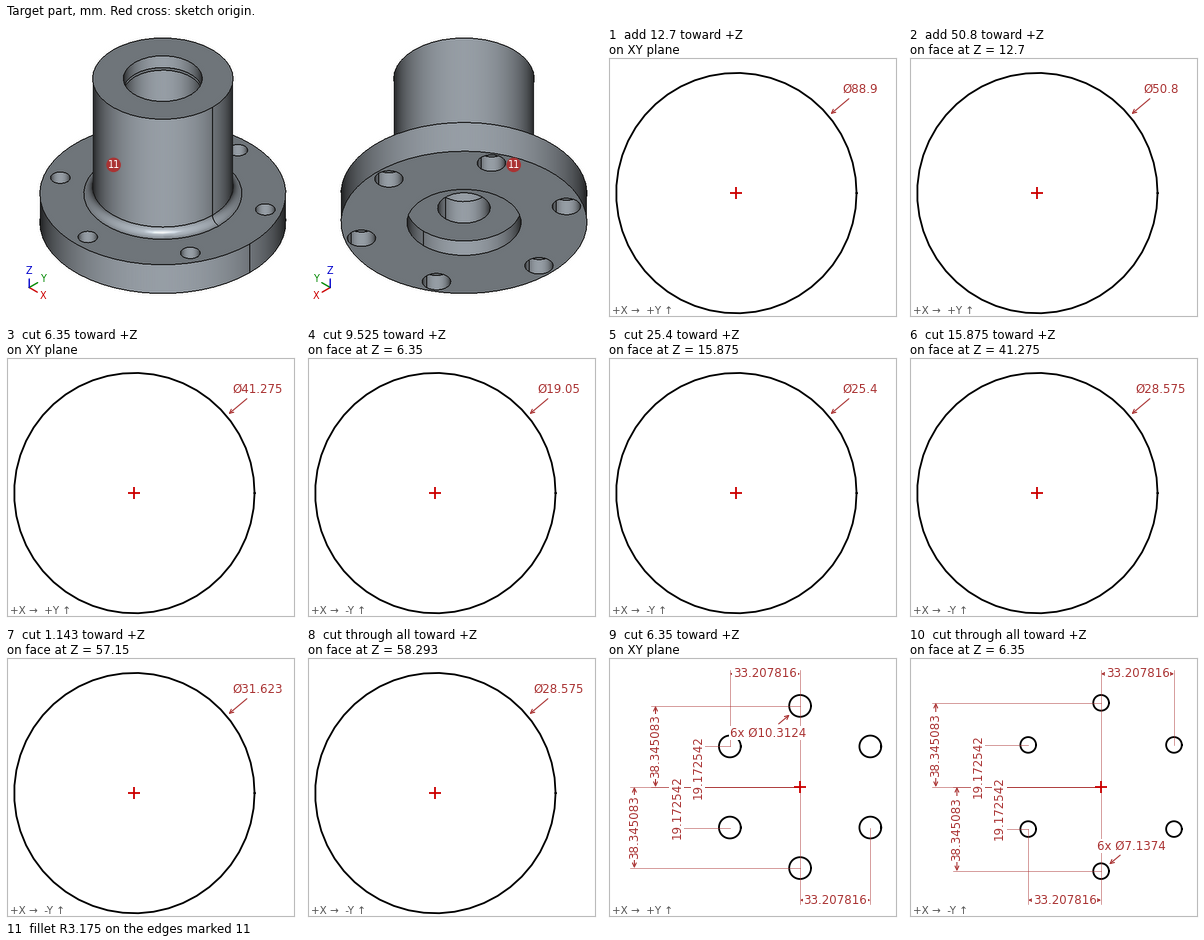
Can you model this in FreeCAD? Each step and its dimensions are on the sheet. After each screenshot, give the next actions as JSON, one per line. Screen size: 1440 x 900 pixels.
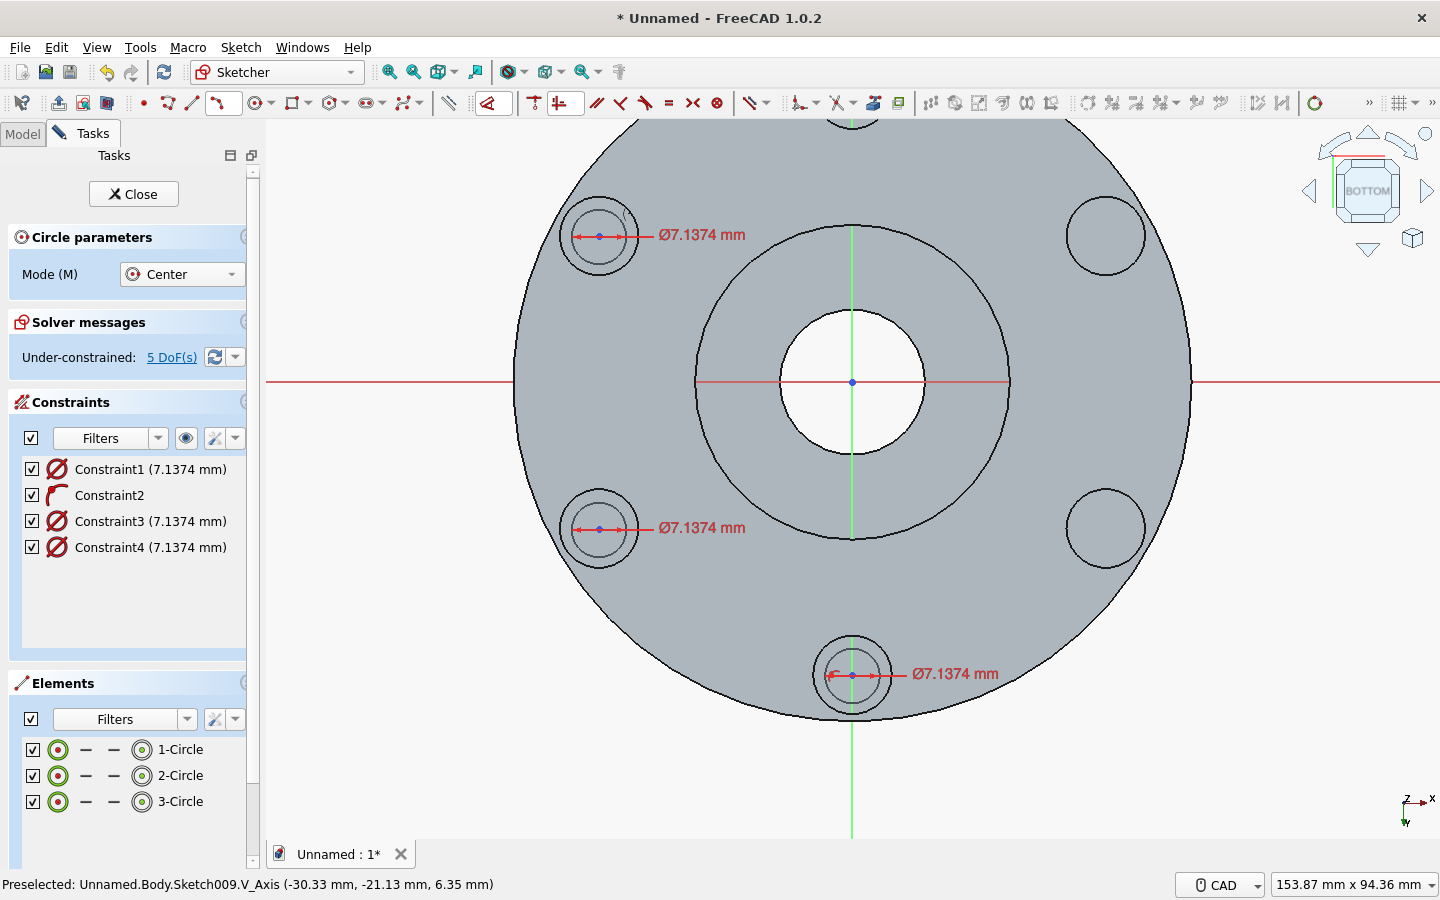
{"action": "scroll", "coordinate": [646, 676], "scroll_direction": "down", "scroll_amount": 2}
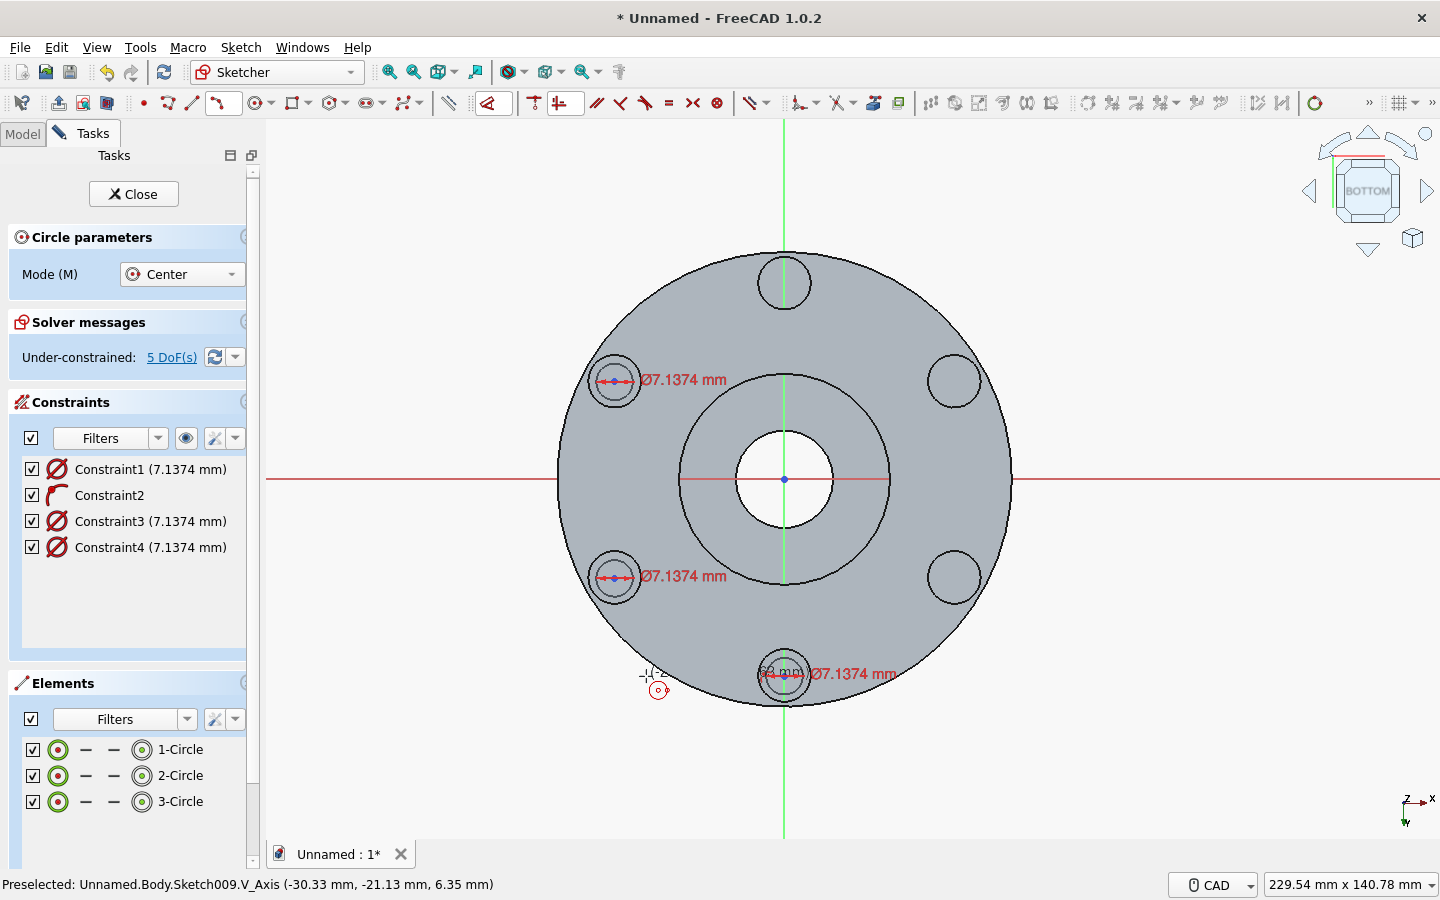
{"action": "scroll", "coordinate": [784, 283], "scroll_direction": "up", "scroll_amount": 2}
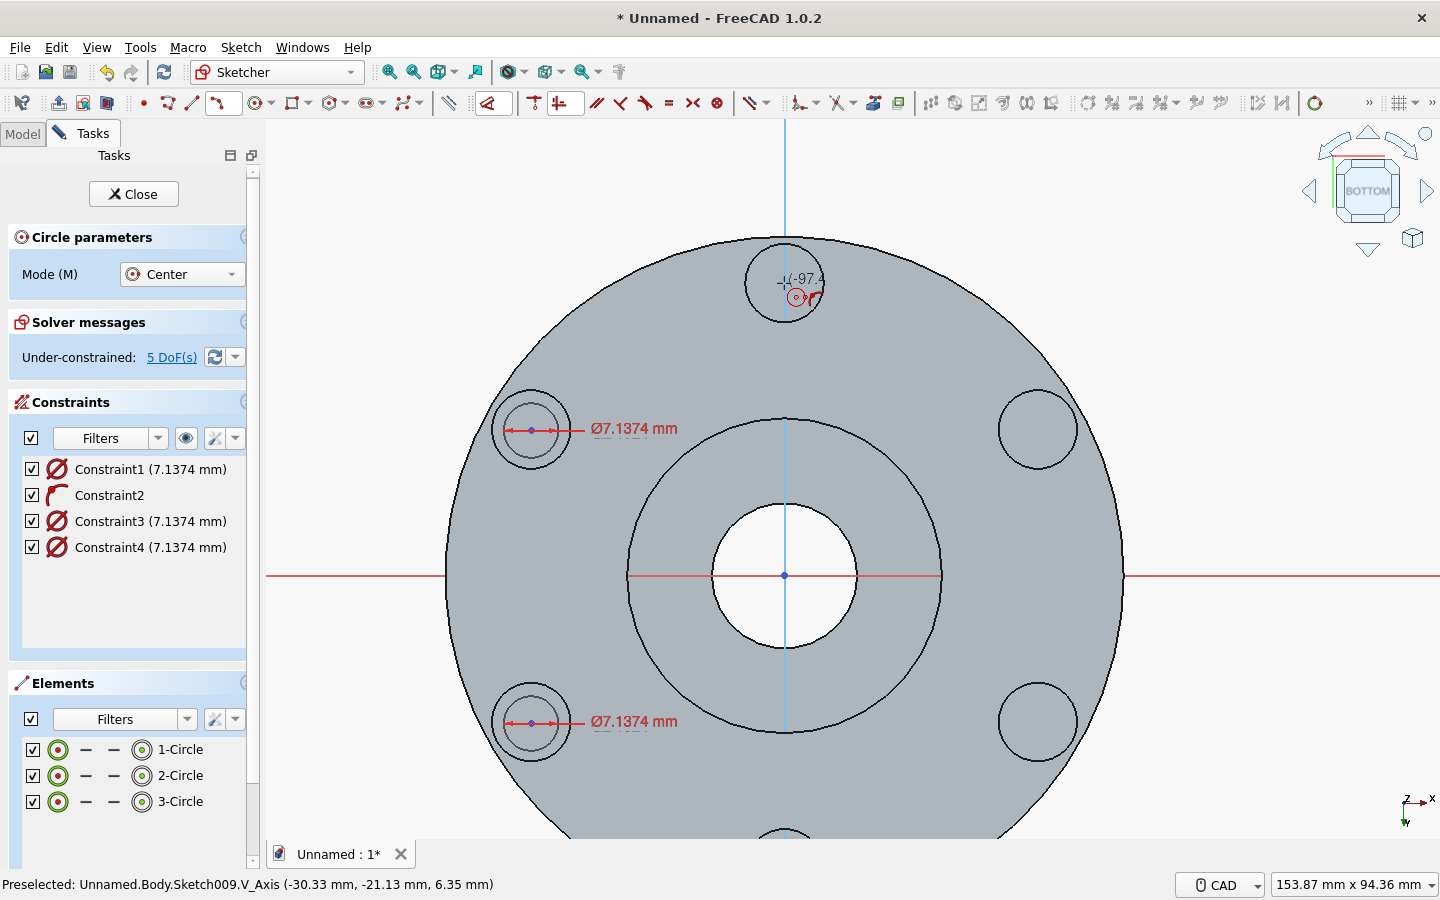
{"action": "left_click", "coordinate": [785, 283]}
{"action": "mouse_move", "coordinate": [804, 264]}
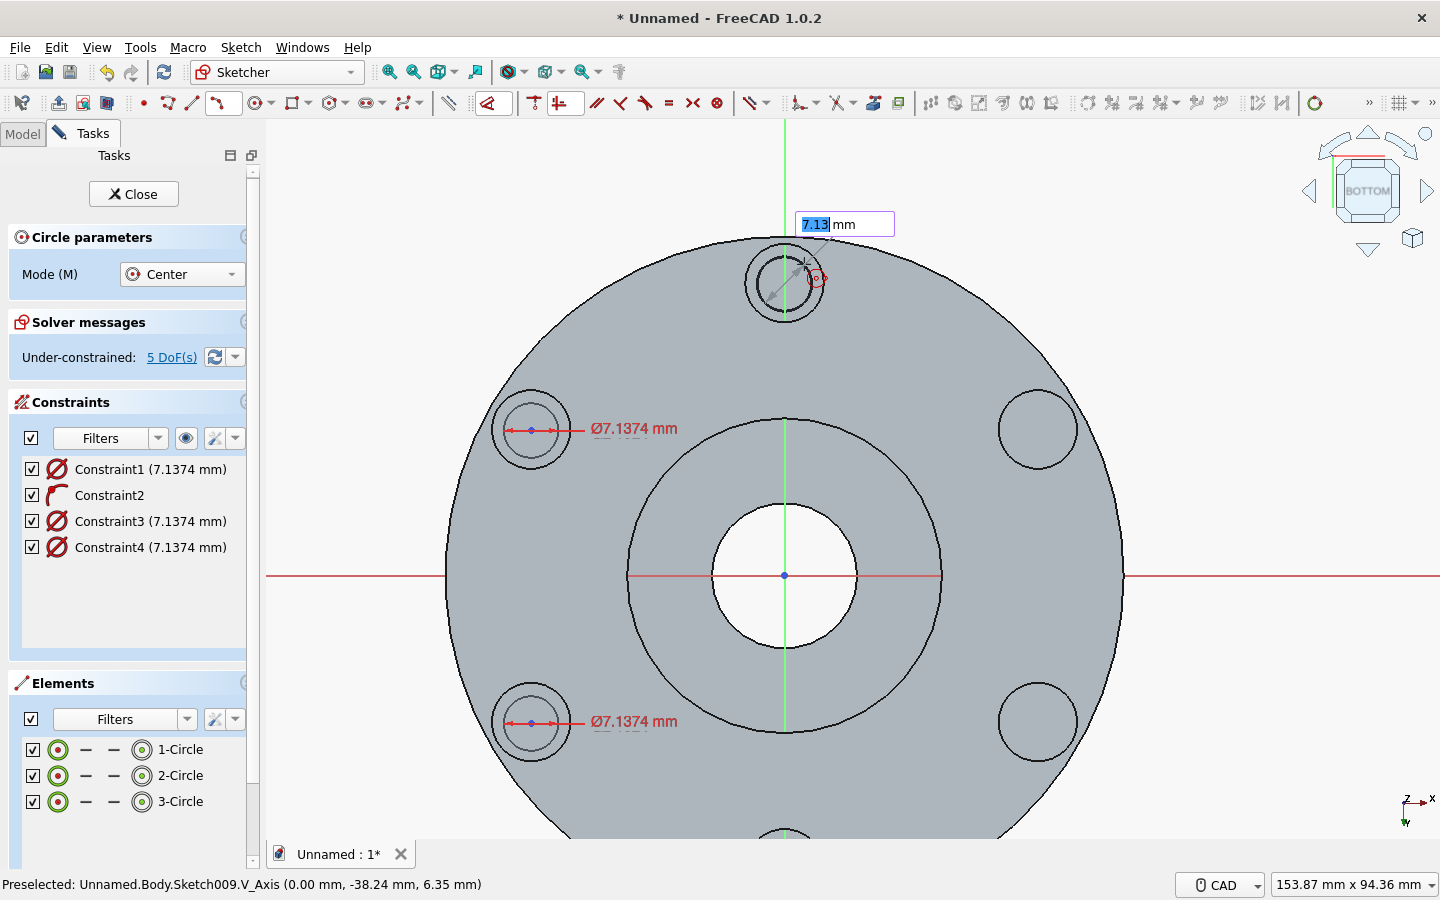
{"action": "type", "text": "7.1374"}
{"action": "key", "text": "Return"}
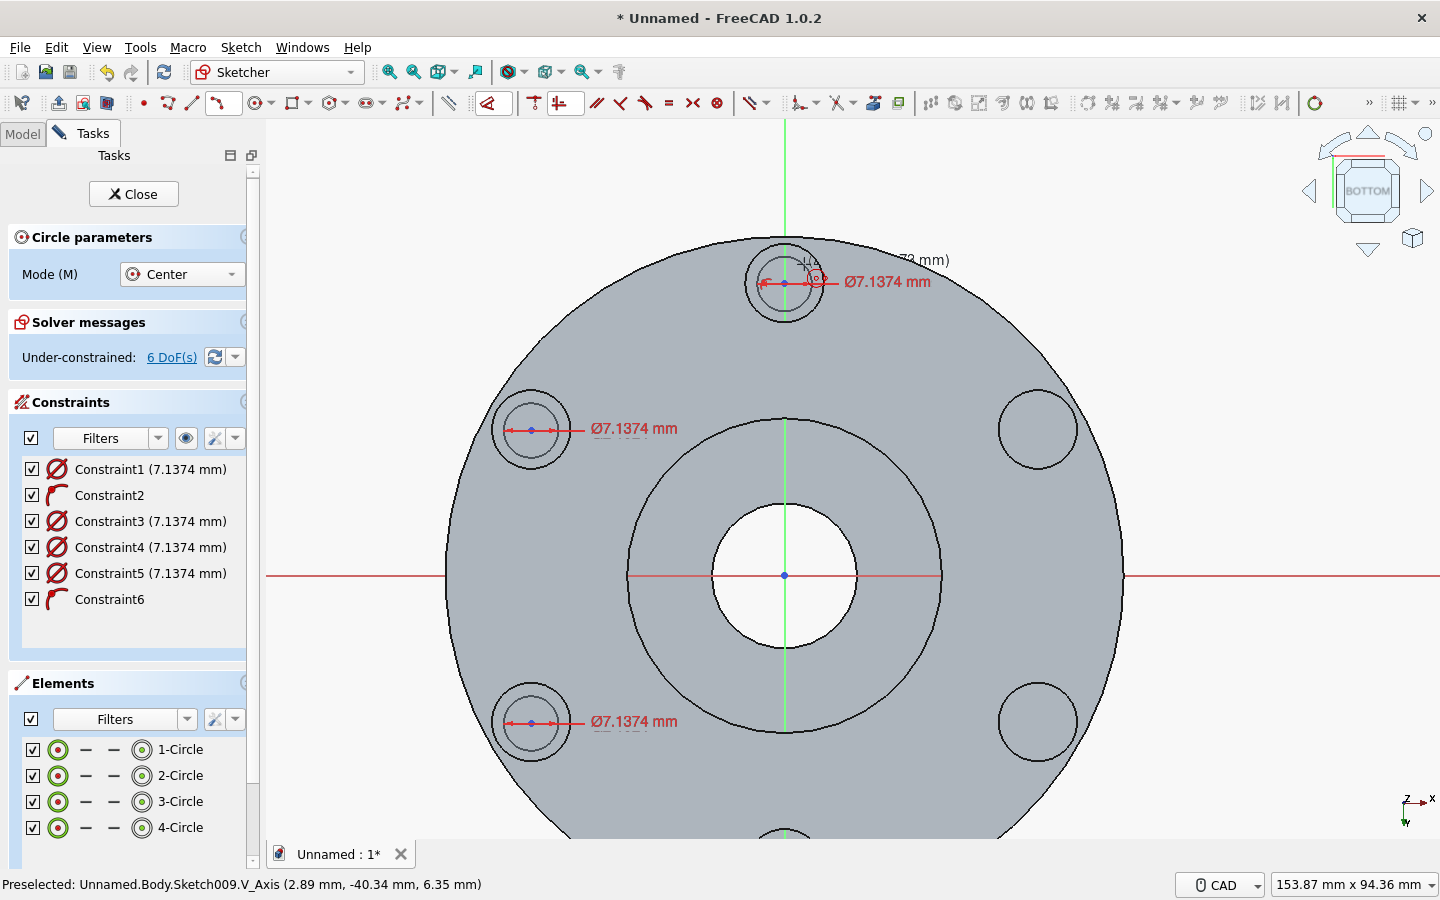
{"action": "left_click", "coordinate": [1038, 429]}
{"action": "mouse_move", "coordinate": [1057, 410]}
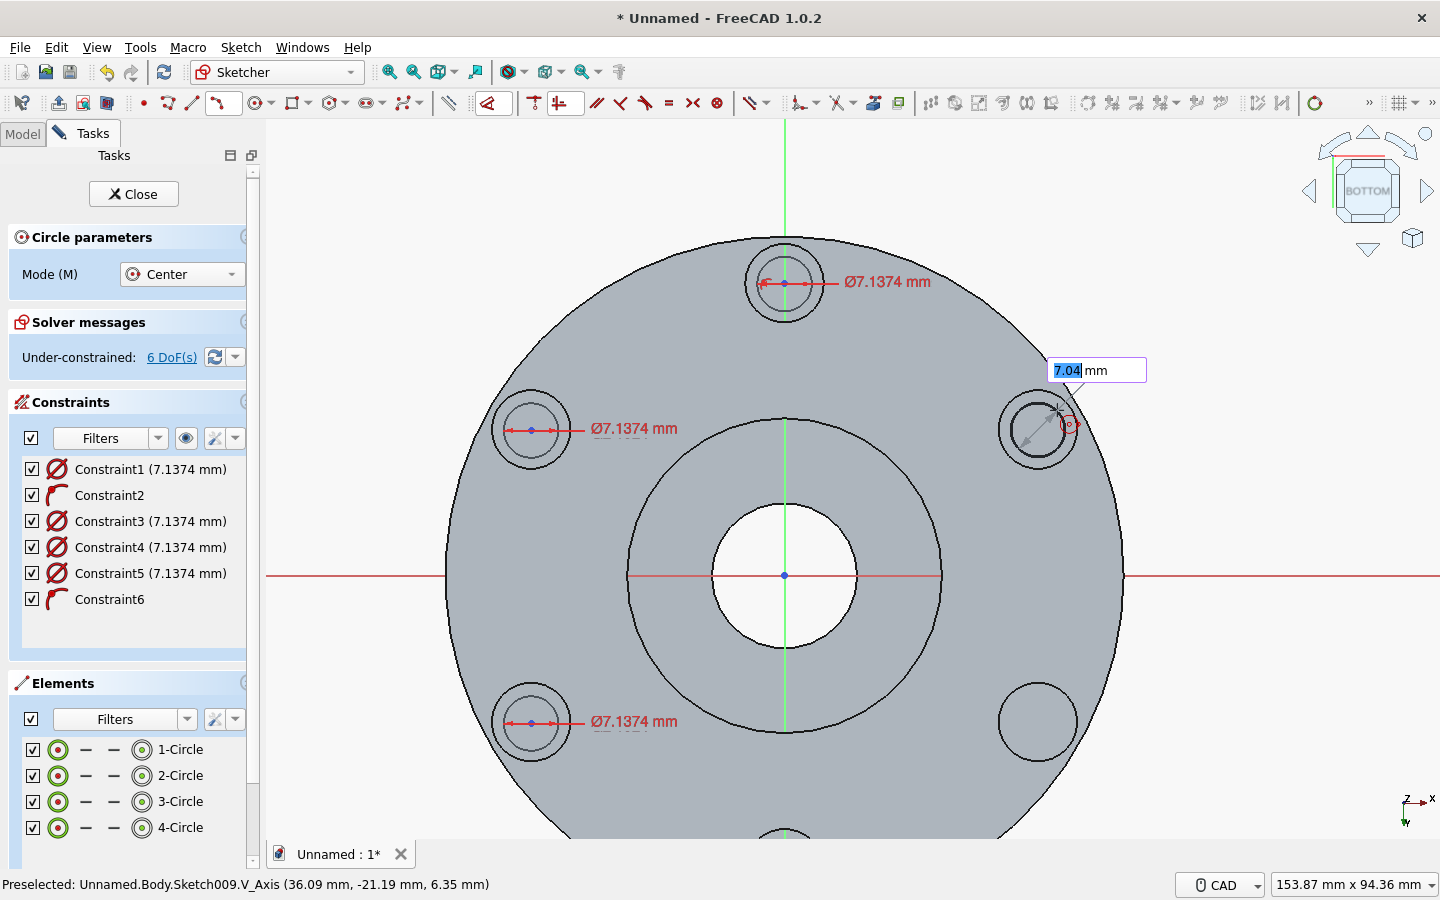
{"action": "type", "text": "7.1374"}
{"action": "key", "text": "Return"}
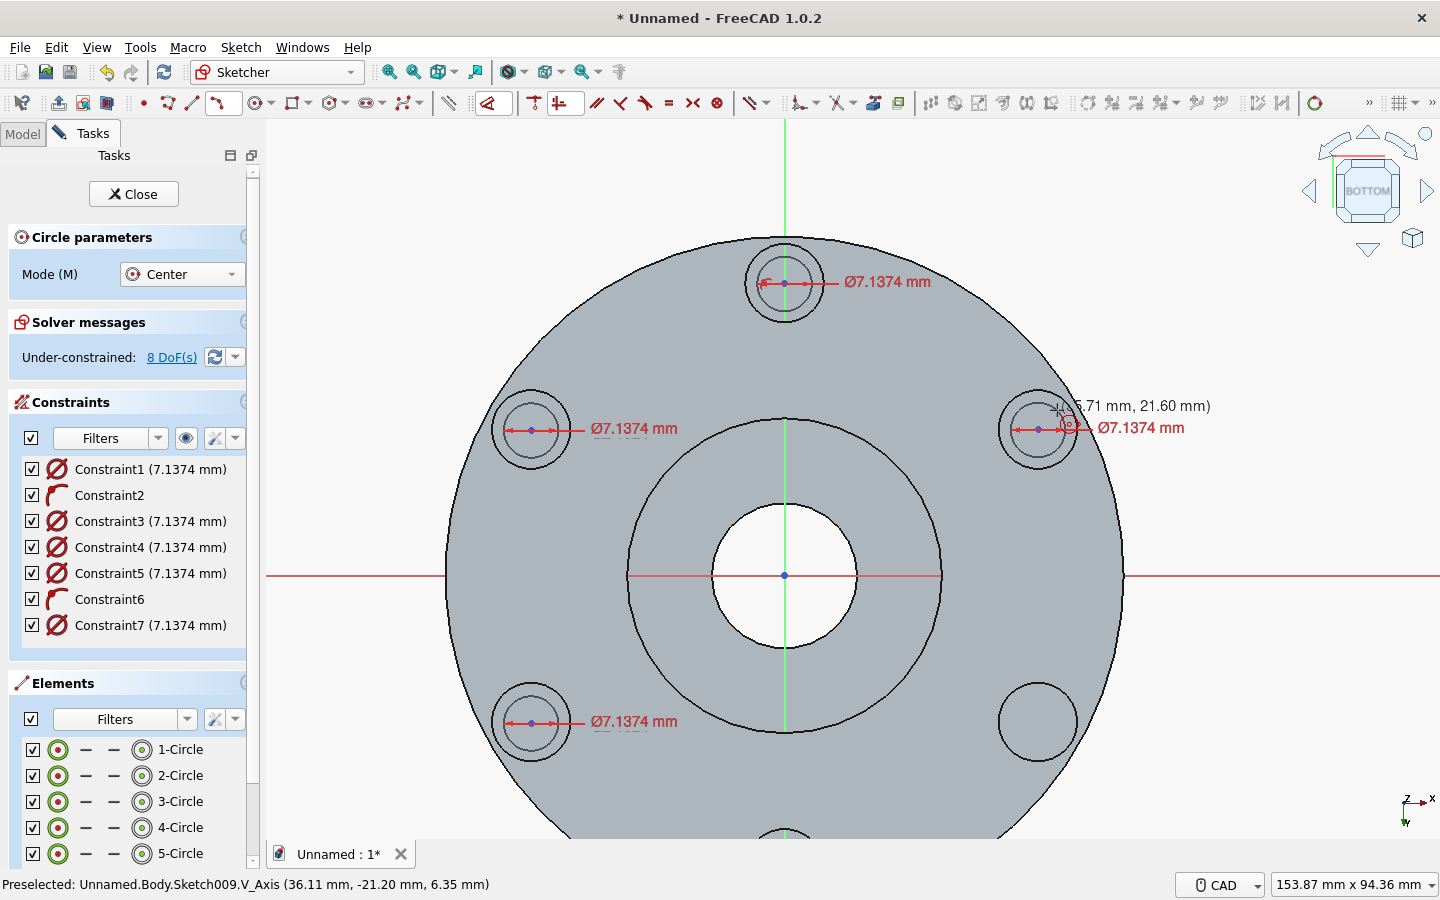
{"action": "left_click", "coordinate": [1038, 722]}
{"action": "mouse_move", "coordinate": [1057, 703]}